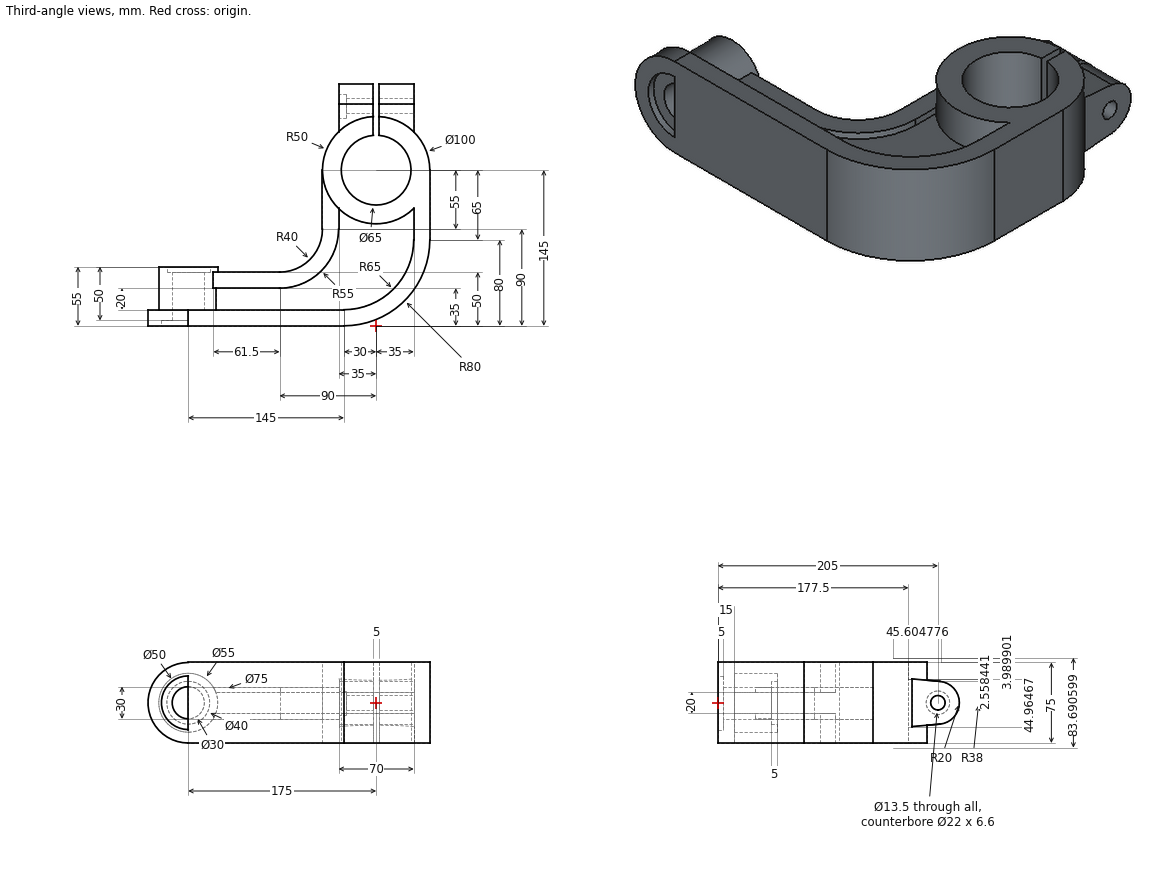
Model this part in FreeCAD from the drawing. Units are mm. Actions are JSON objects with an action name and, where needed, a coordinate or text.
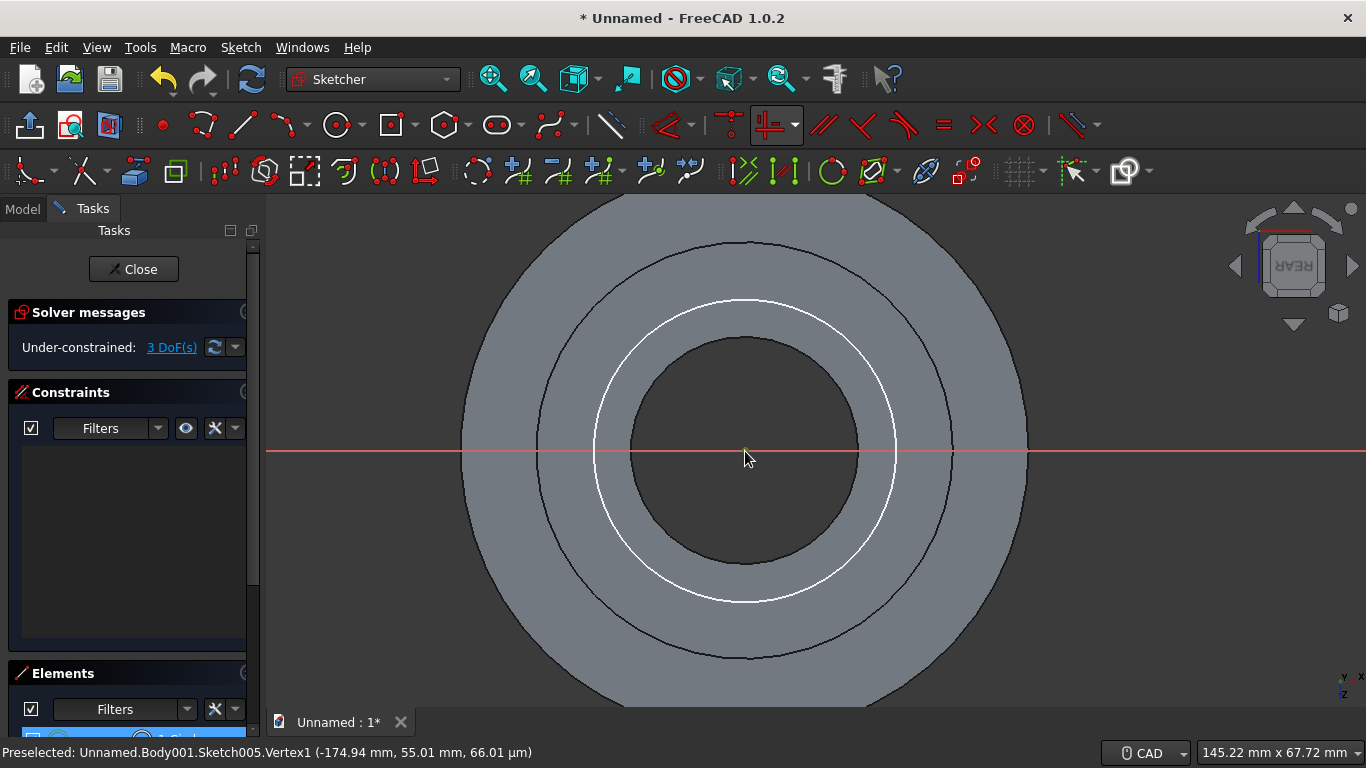
{"action": "left_click", "coordinate": [359, 450]}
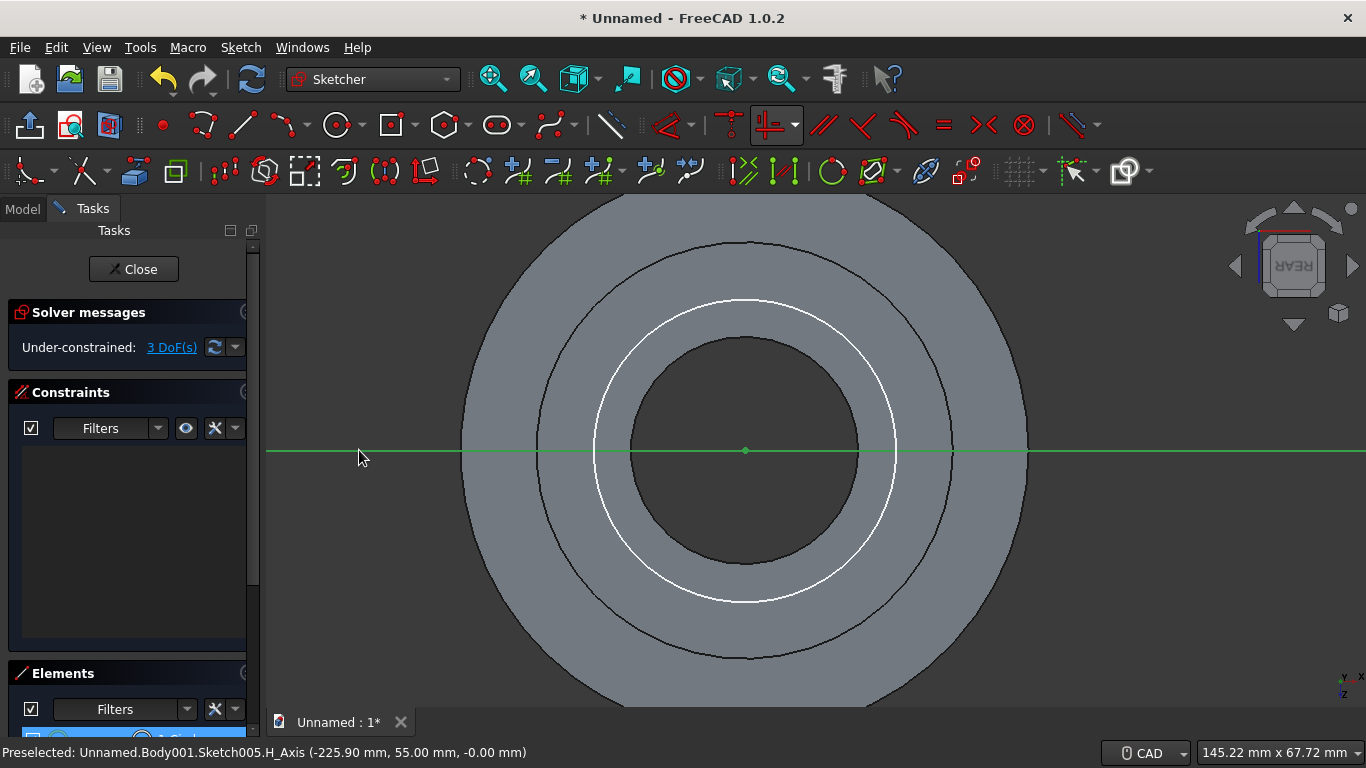
{"action": "key", "text": "c"}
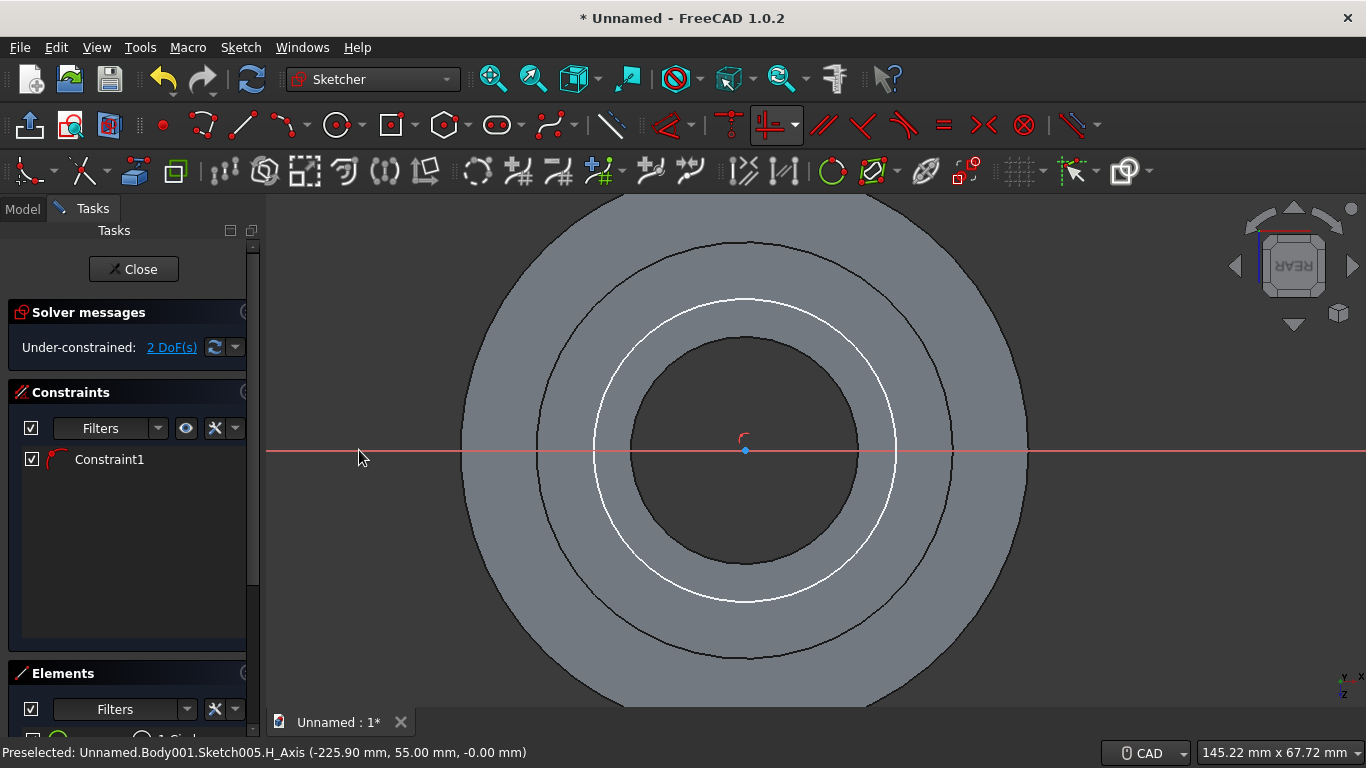
{"action": "key", "text": "d"}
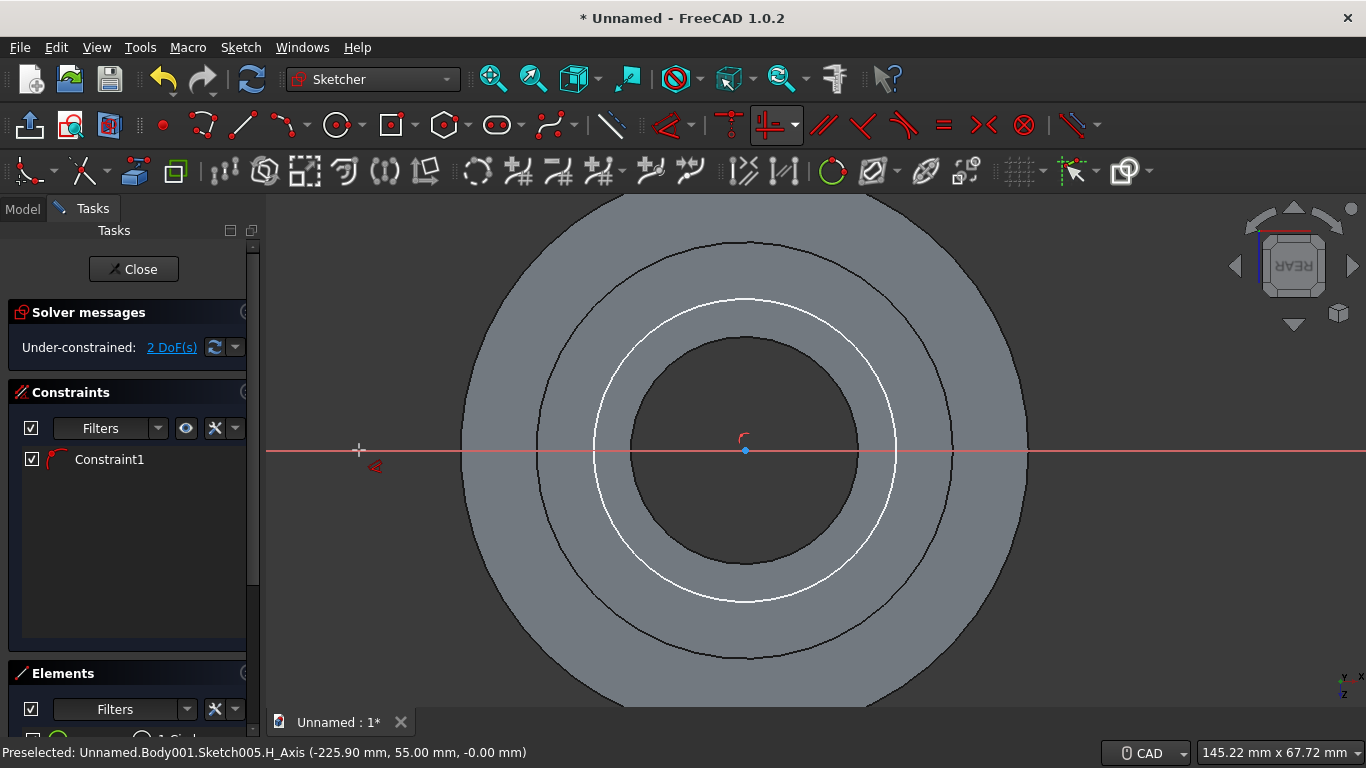
{"action": "left_click", "coordinate": [852, 343]}
{"action": "left_click", "coordinate": [875, 320]}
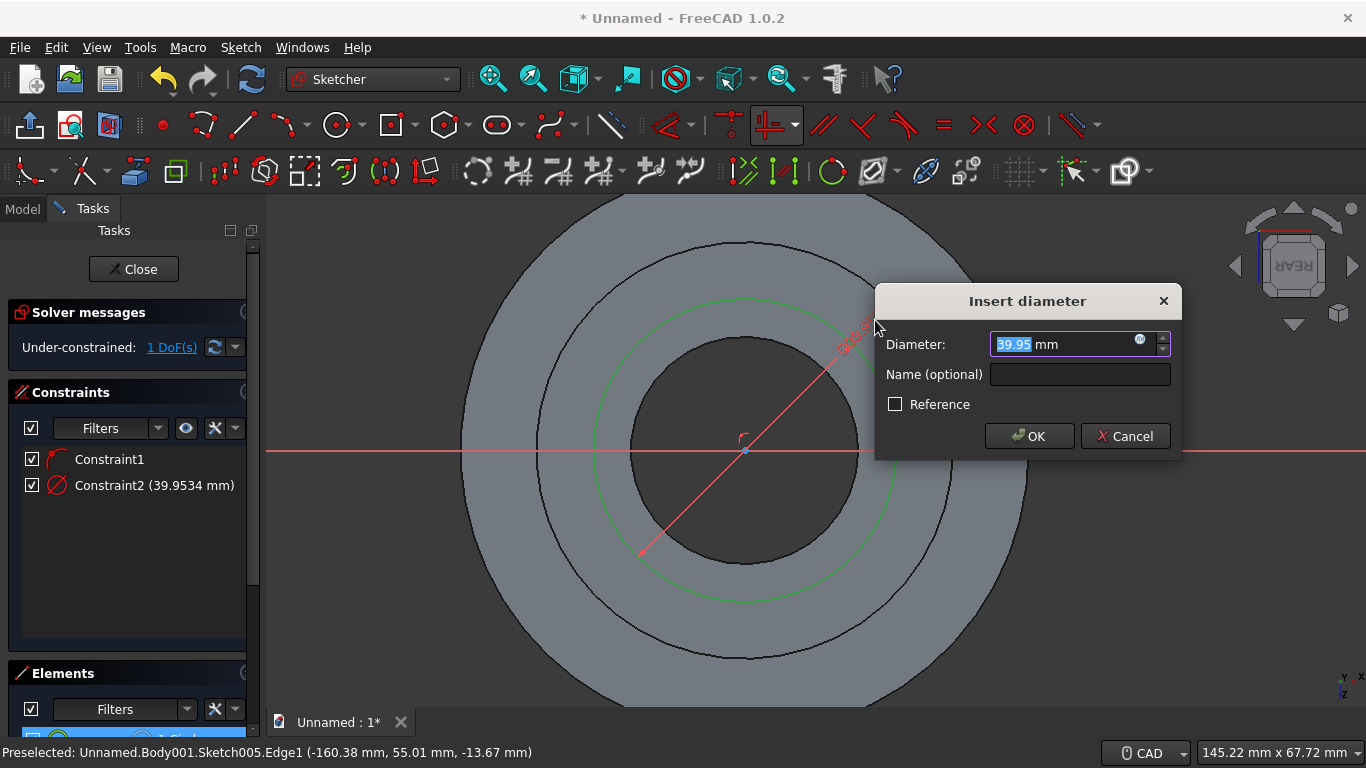
{"action": "type", "text": "40"}
{"action": "key", "text": "Return"}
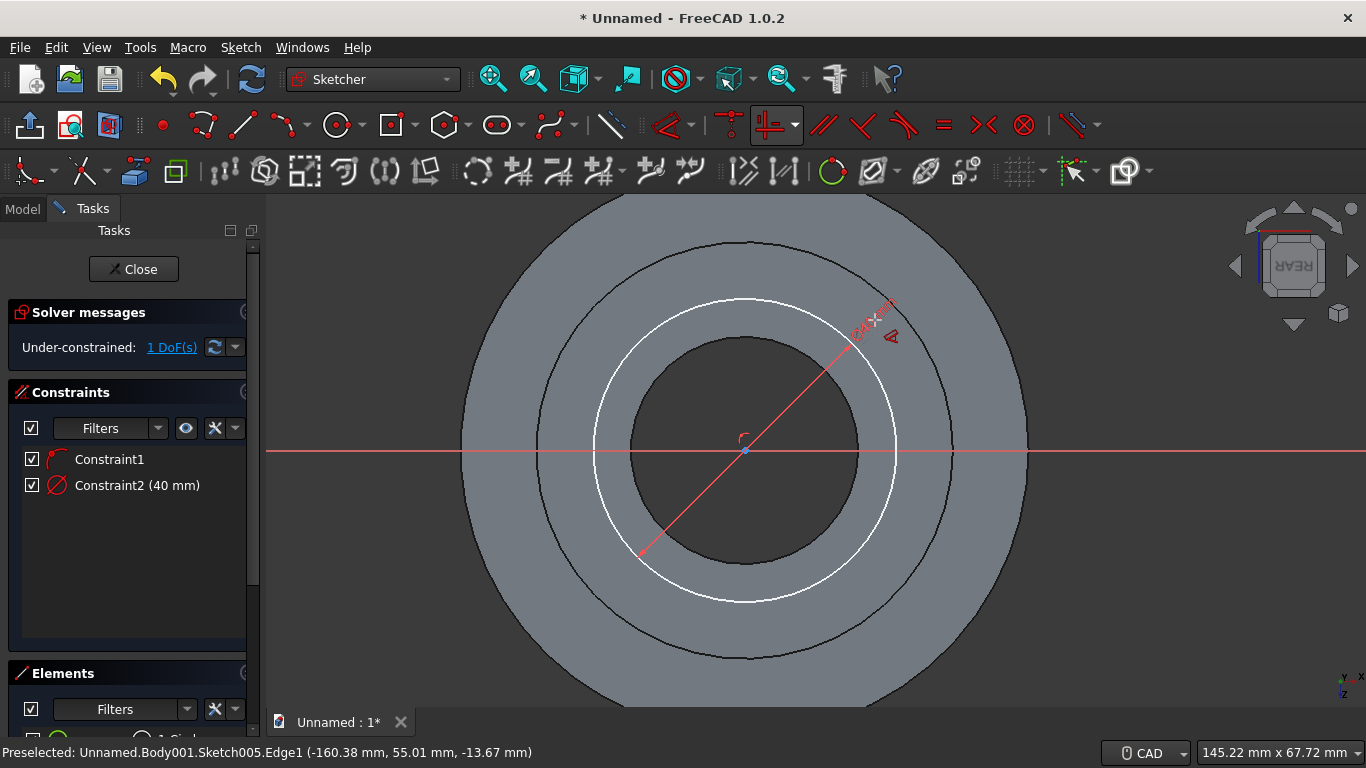
{"action": "left_click", "coordinate": [745, 450]}
{"action": "left_click", "coordinate": [973, 484]}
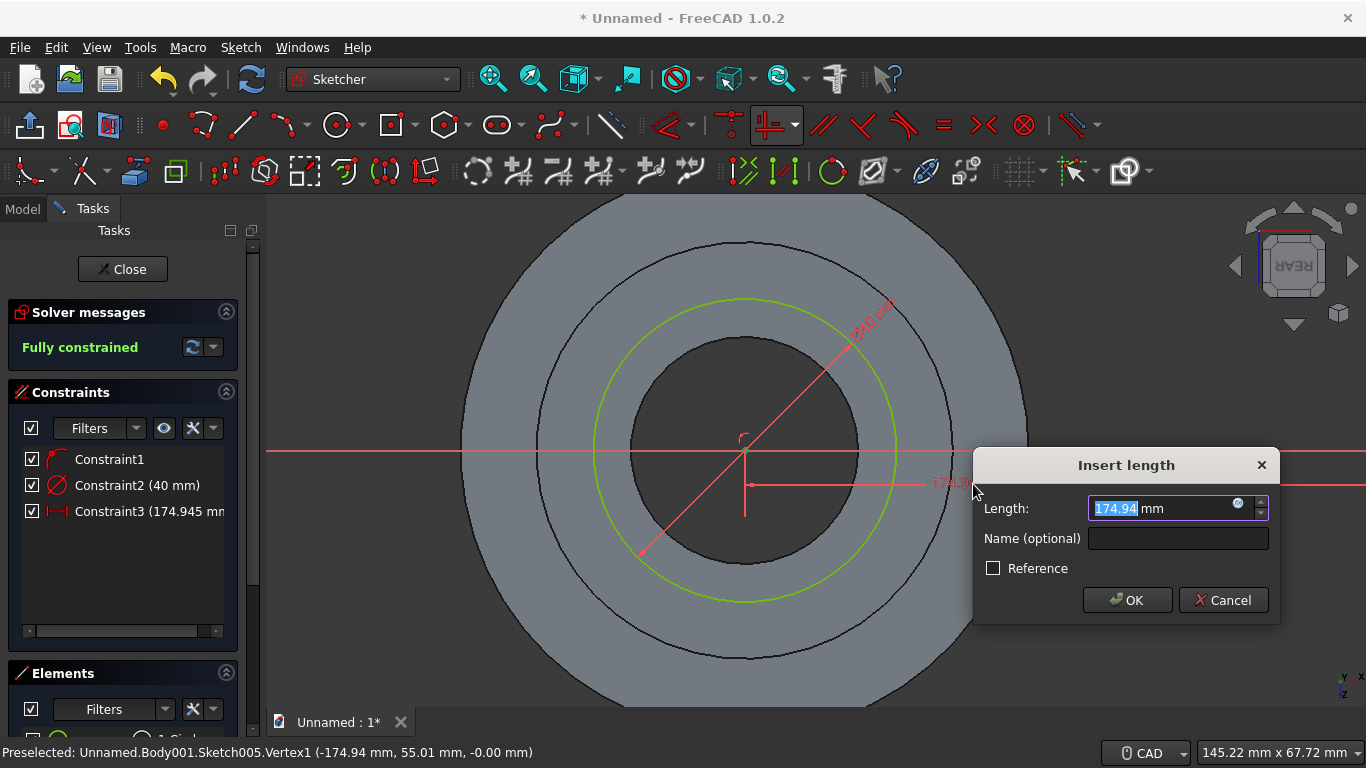
{"action": "type", "text": "175"}
{"action": "key", "text": "Return"}
{"action": "key", "text": "Escape"}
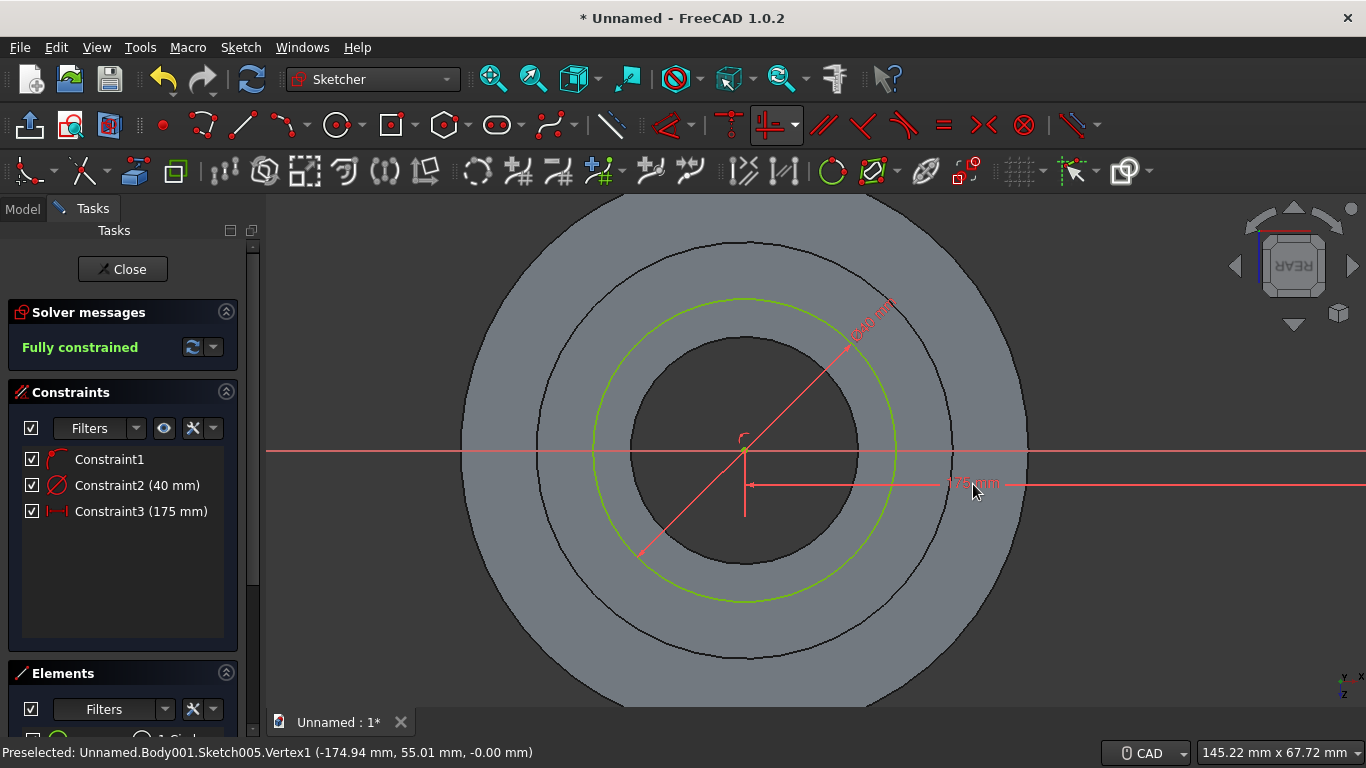
{"action": "left_click", "coordinate": [123, 269]}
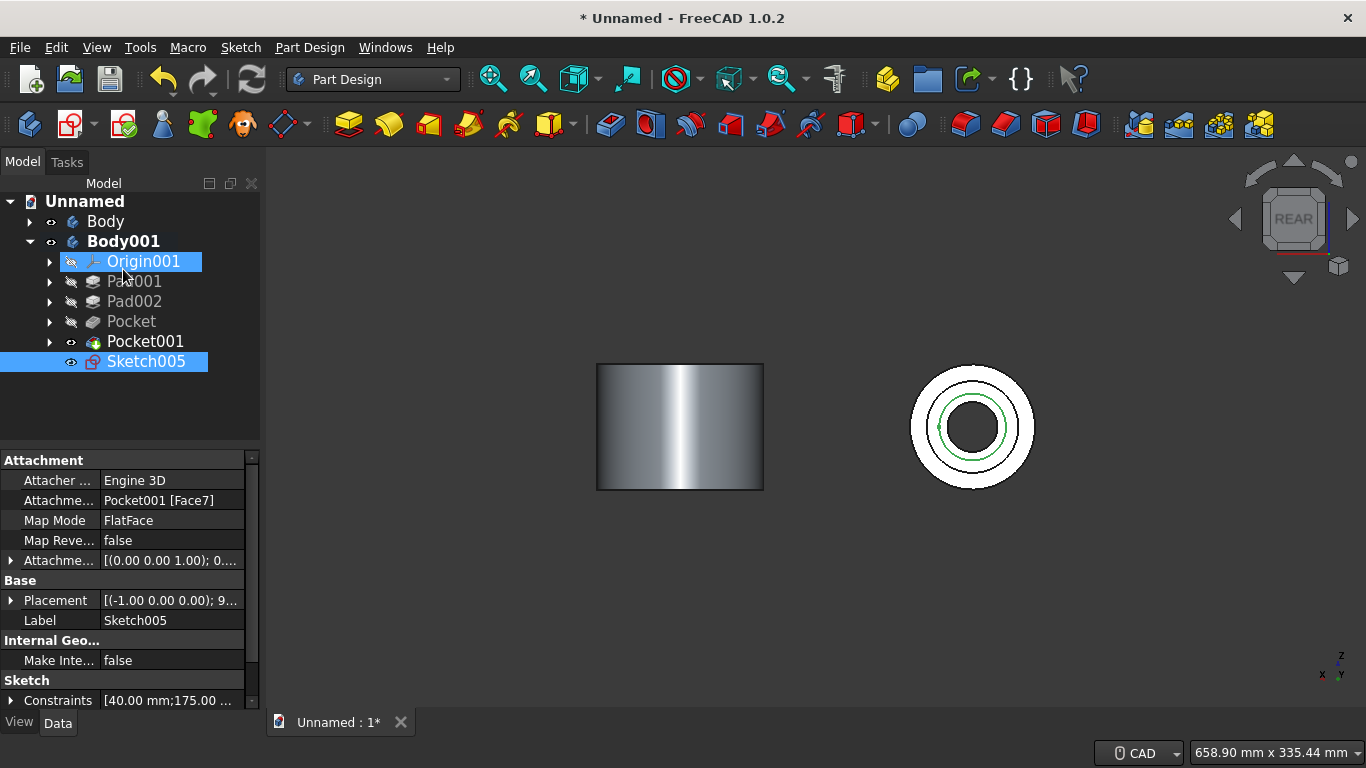
{"action": "left_click", "coordinate": [612, 124]}